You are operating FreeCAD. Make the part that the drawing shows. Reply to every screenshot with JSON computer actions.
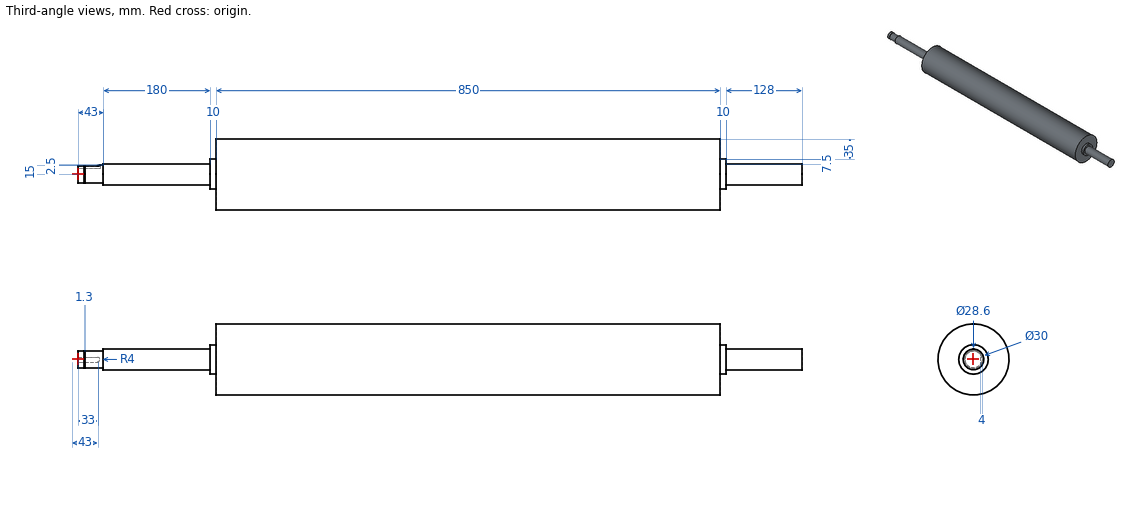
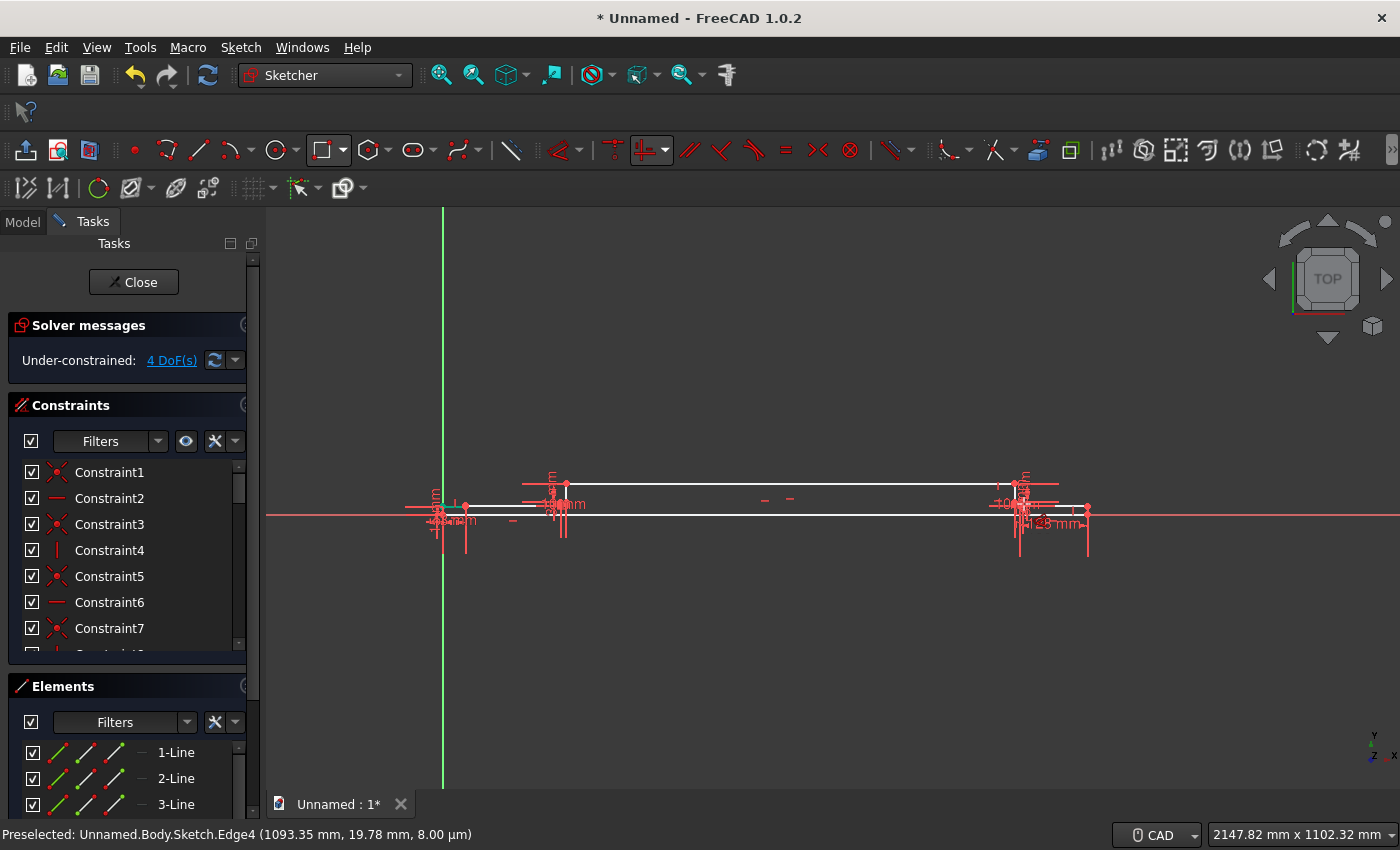
{"action": "left_click", "coordinate": [880, 484]}
{"action": "left_click", "coordinate": [791, 450]}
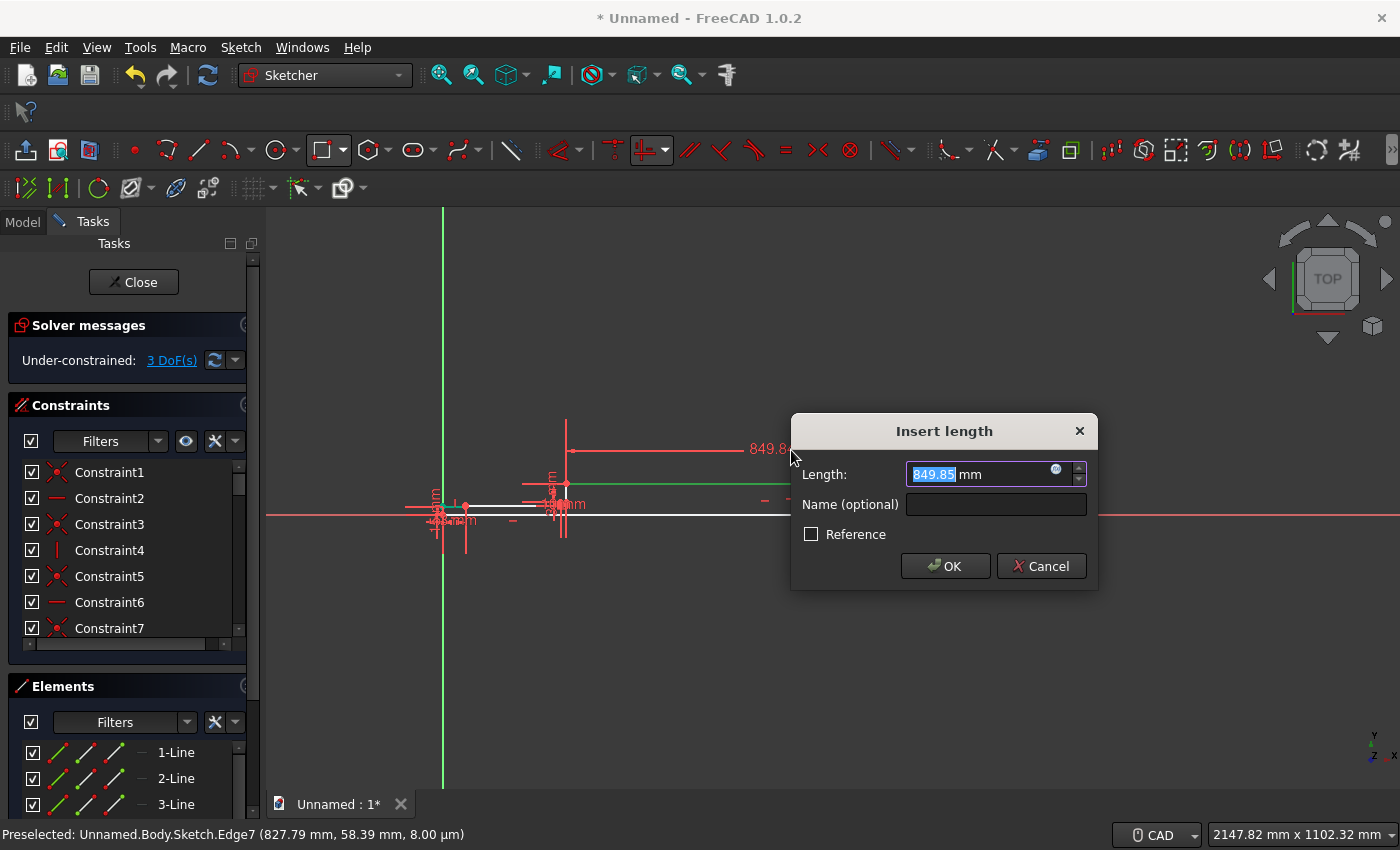
{"action": "type", "text": "850"}
{"action": "key", "text": "Return"}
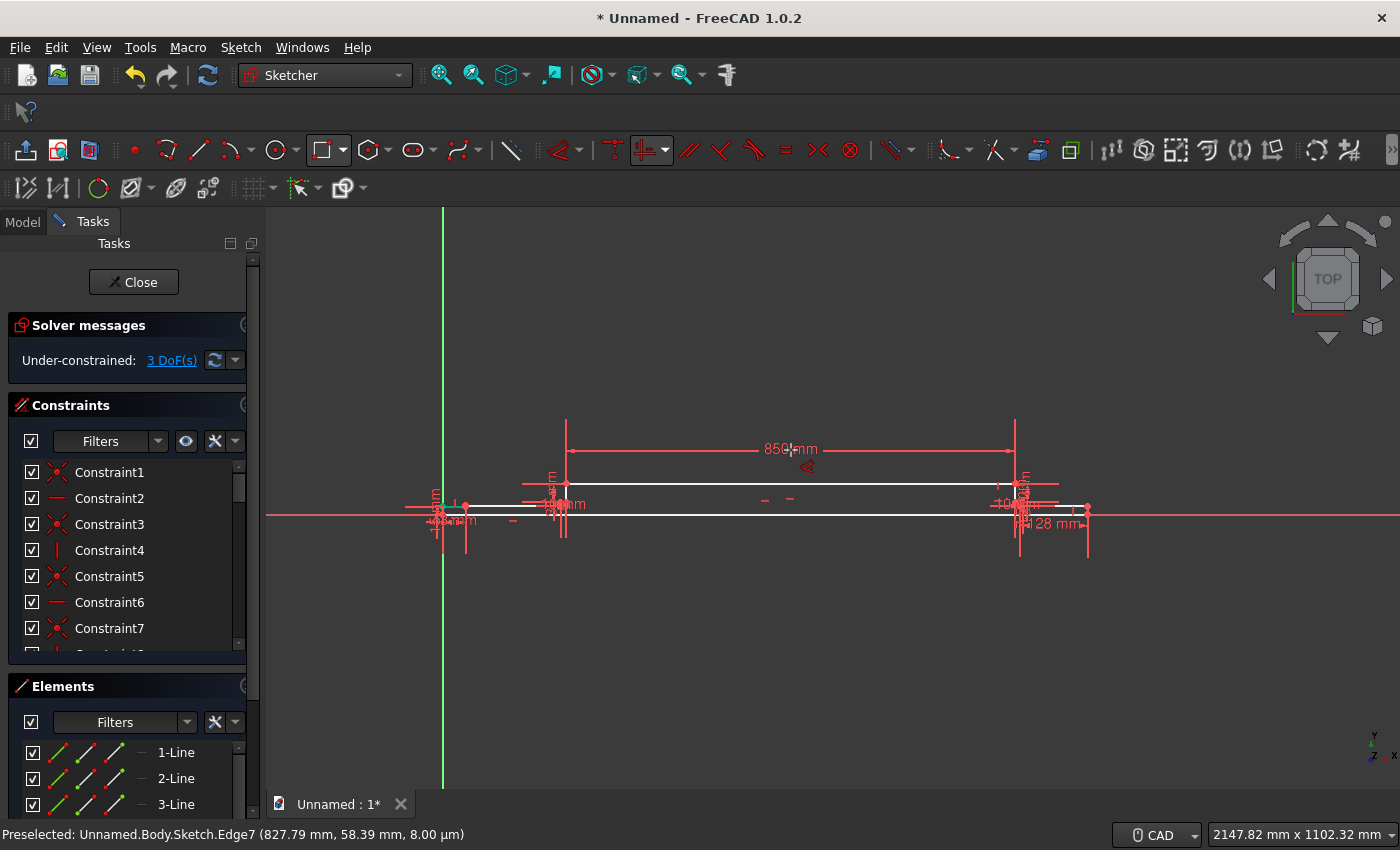
{"action": "scroll", "coordinate": [561, 504], "scroll_direction": "up", "scroll_amount": 12}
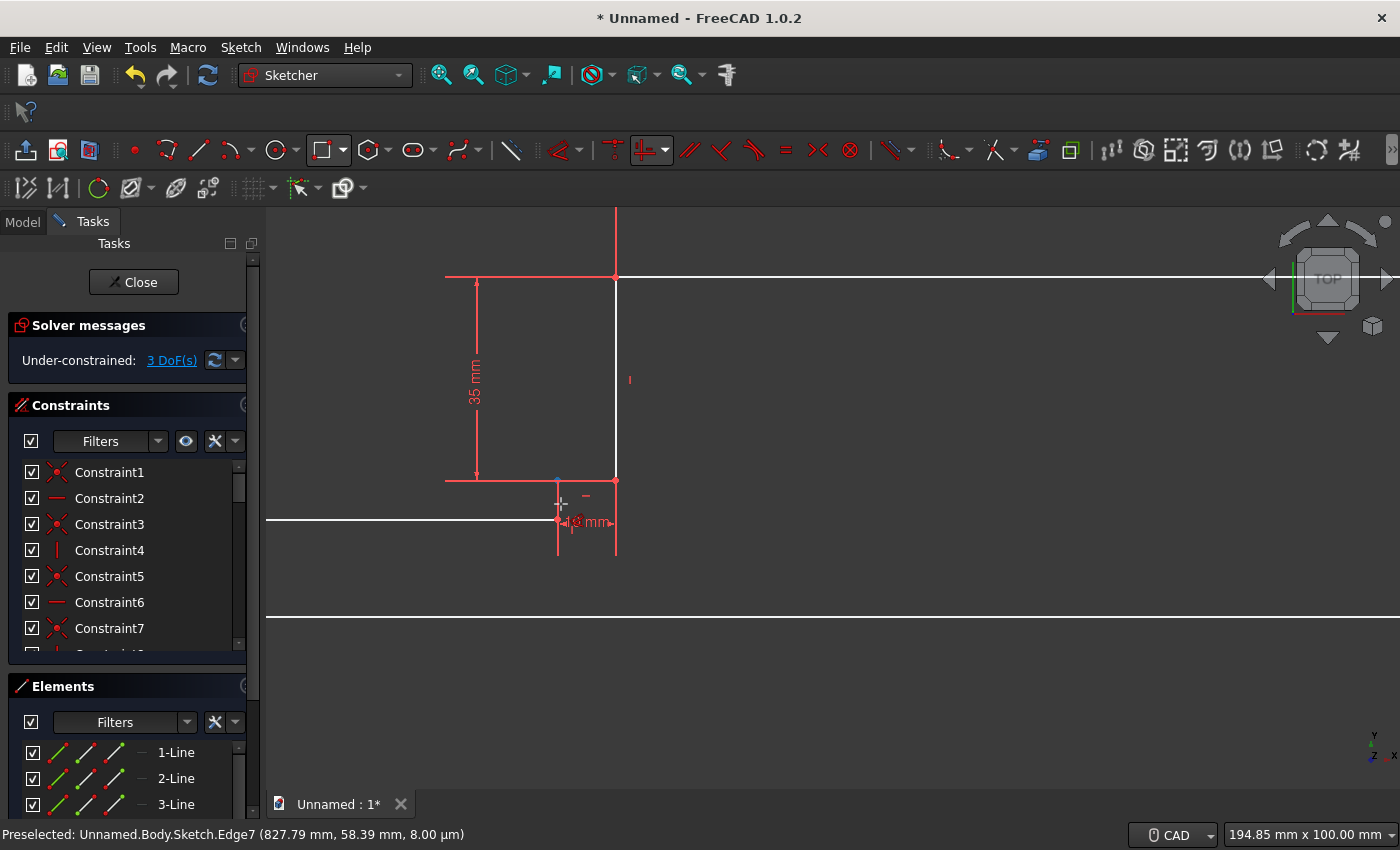
{"action": "left_click", "coordinate": [558, 500]}
{"action": "left_click", "coordinate": [524, 500]}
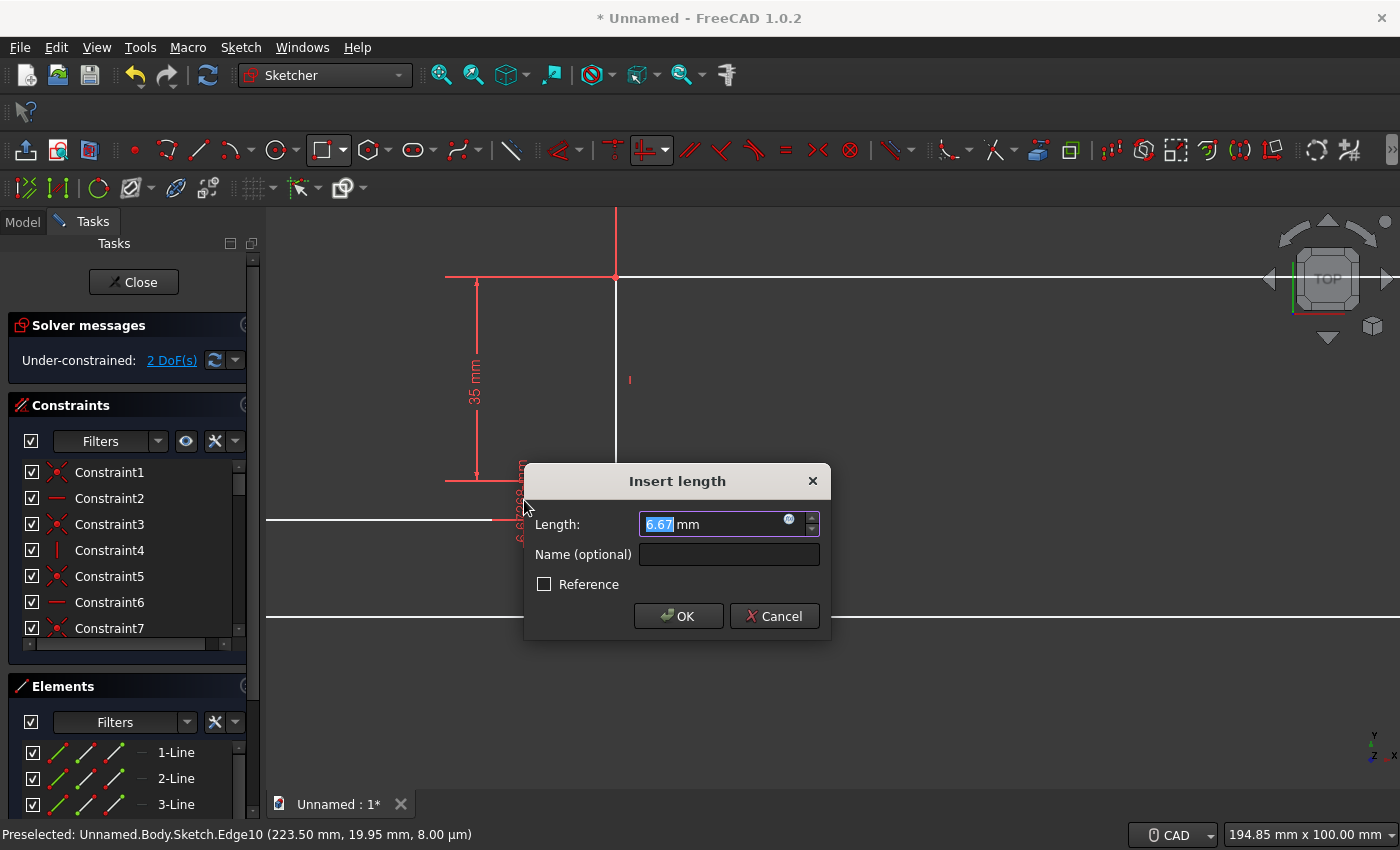
{"action": "type", "text": "7.5"}
{"action": "key", "text": "Return"}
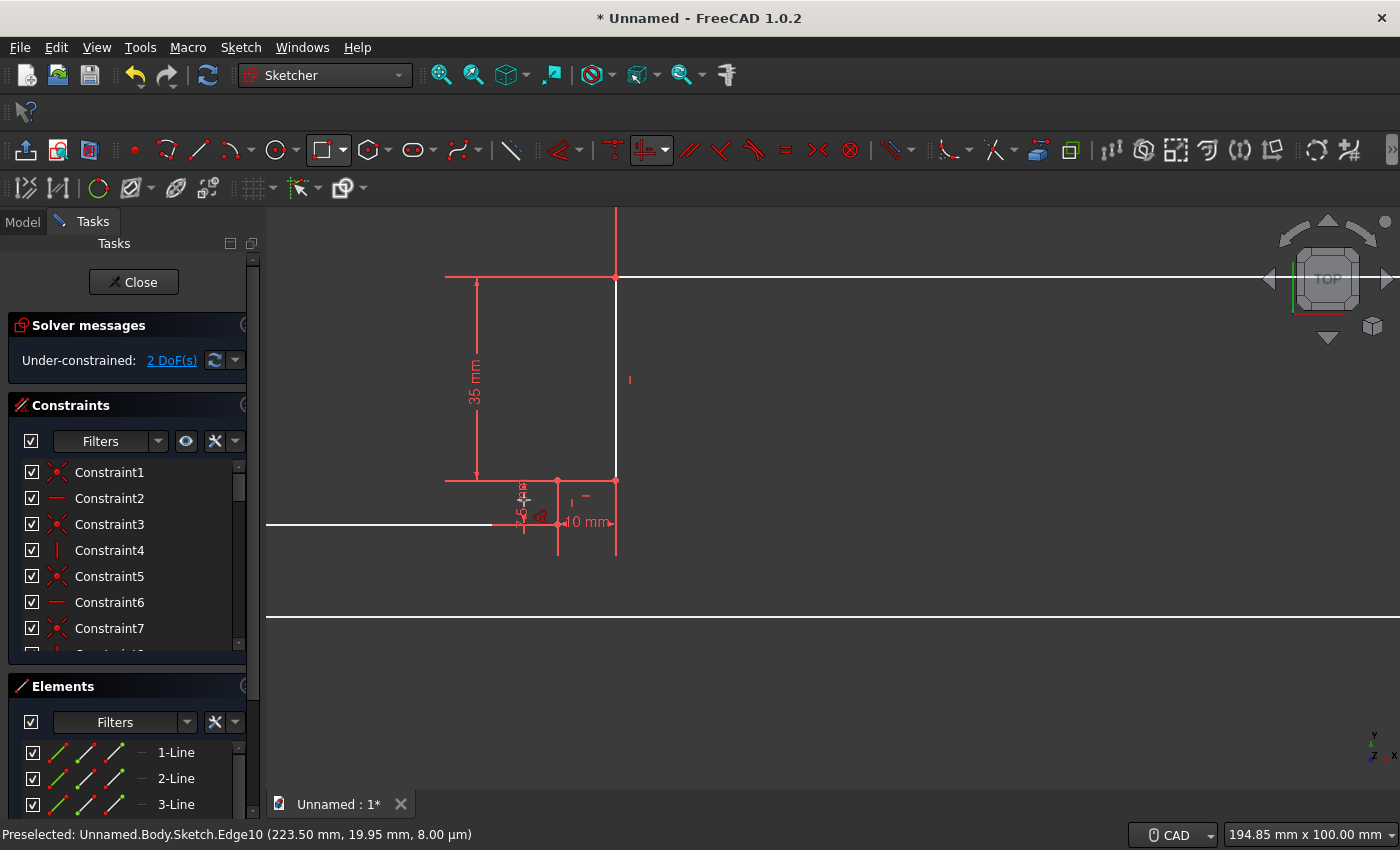
{"action": "scroll", "coordinate": [560, 504], "scroll_direction": "down", "scroll_amount": 12}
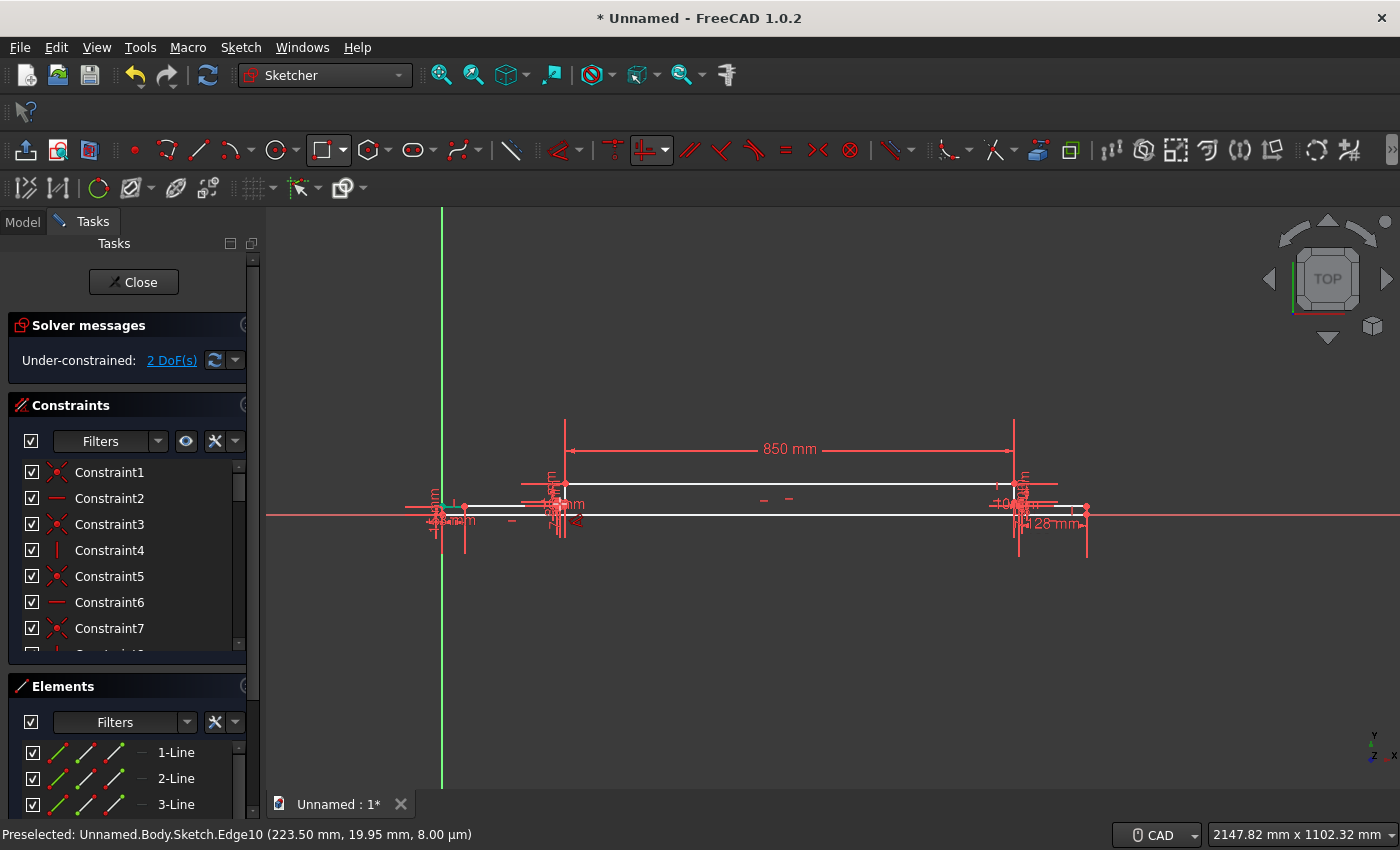
{"action": "scroll", "coordinate": [541, 506], "scroll_direction": "up", "scroll_amount": 3}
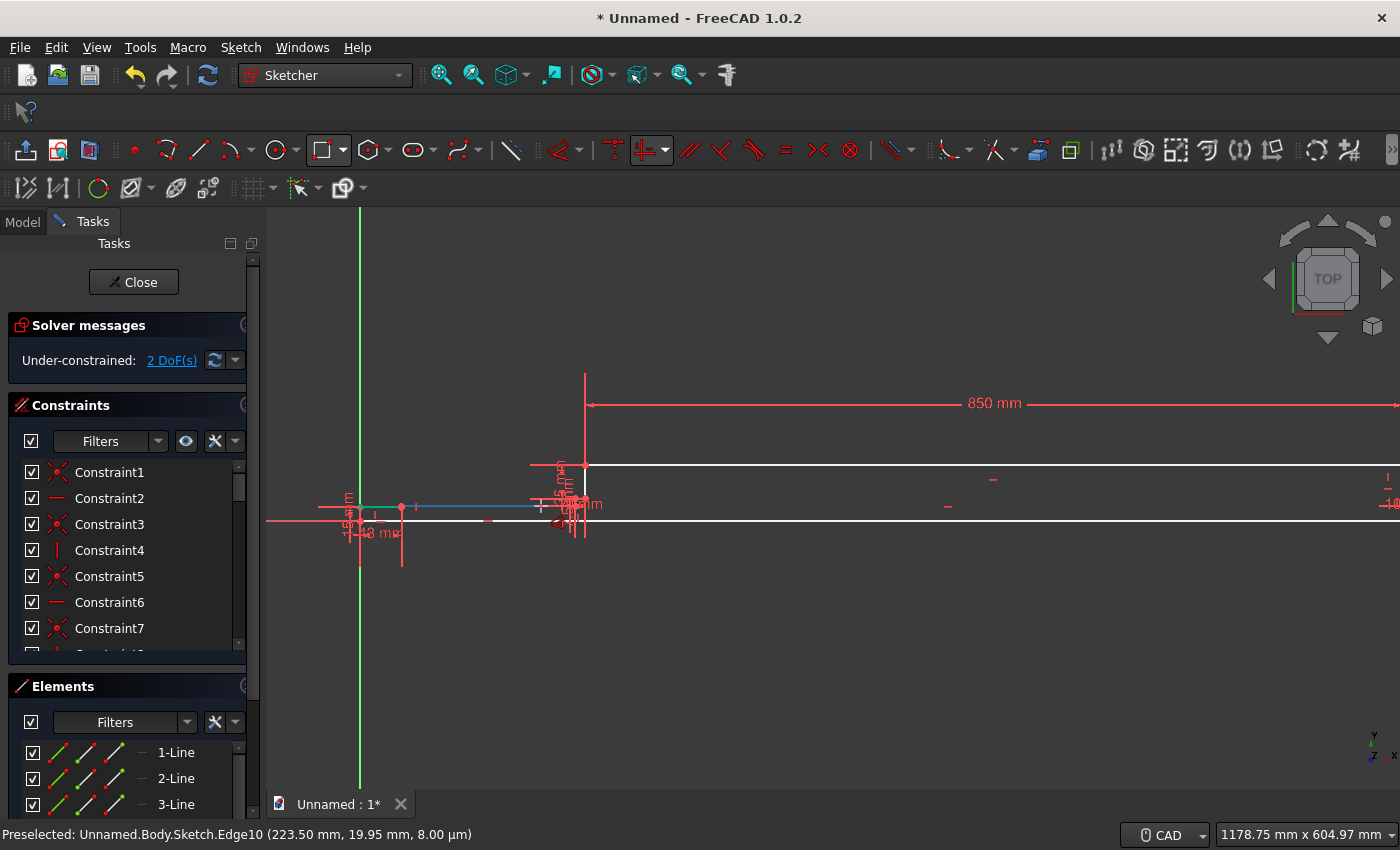
{"action": "left_click", "coordinate": [541, 506]}
{"action": "left_click", "coordinate": [489, 540]}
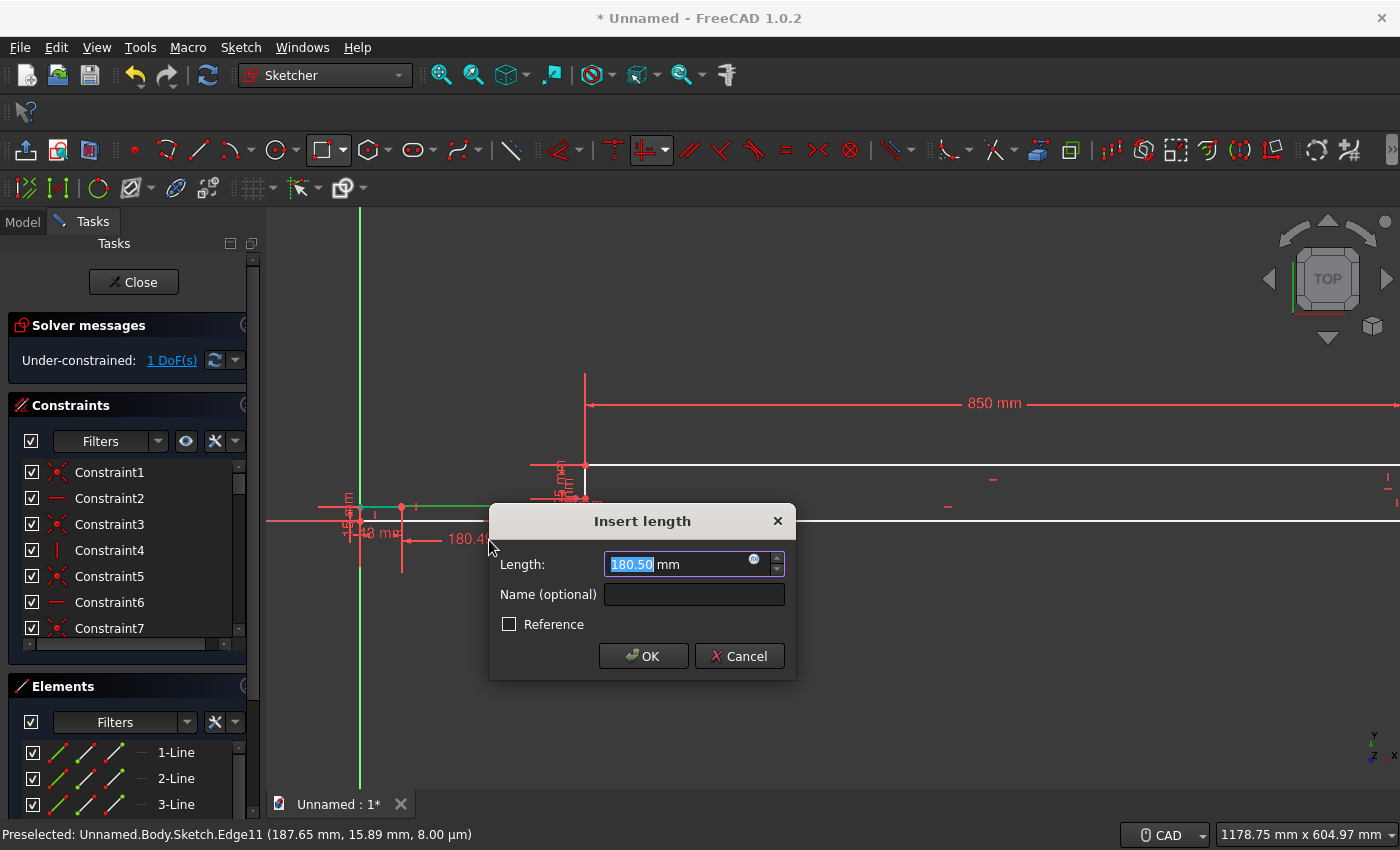
{"action": "type", "text": "180"}
{"action": "key", "text": "Return"}